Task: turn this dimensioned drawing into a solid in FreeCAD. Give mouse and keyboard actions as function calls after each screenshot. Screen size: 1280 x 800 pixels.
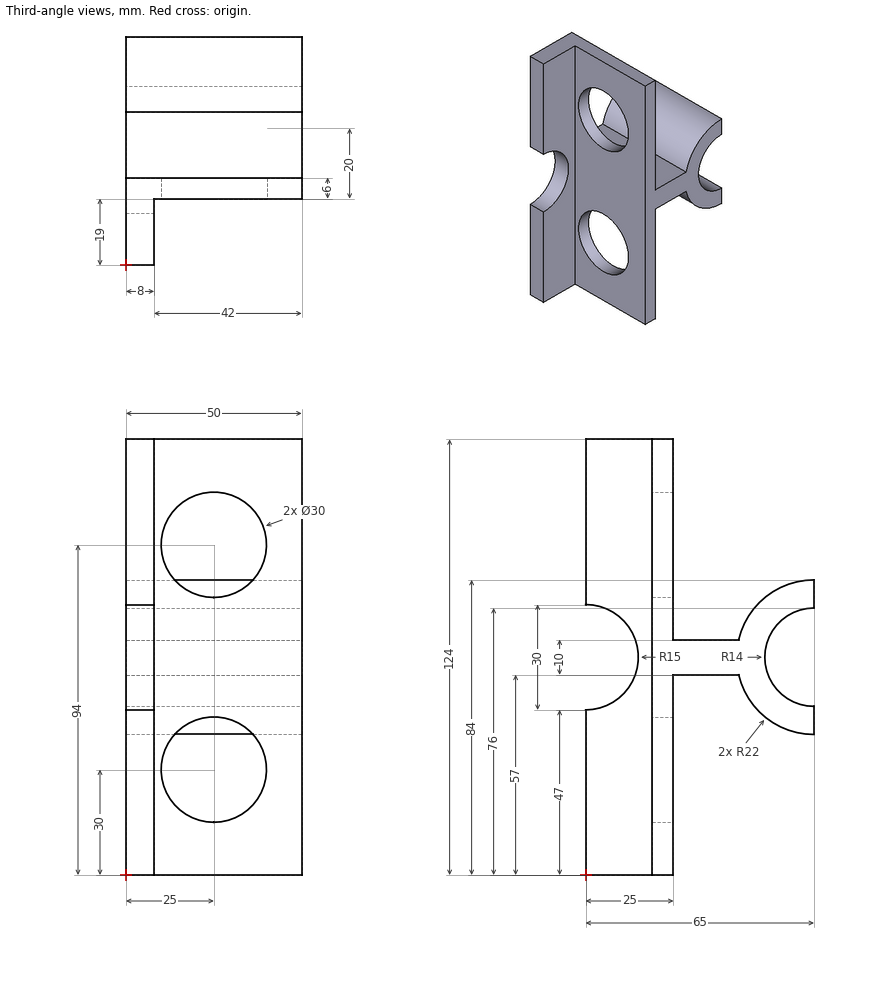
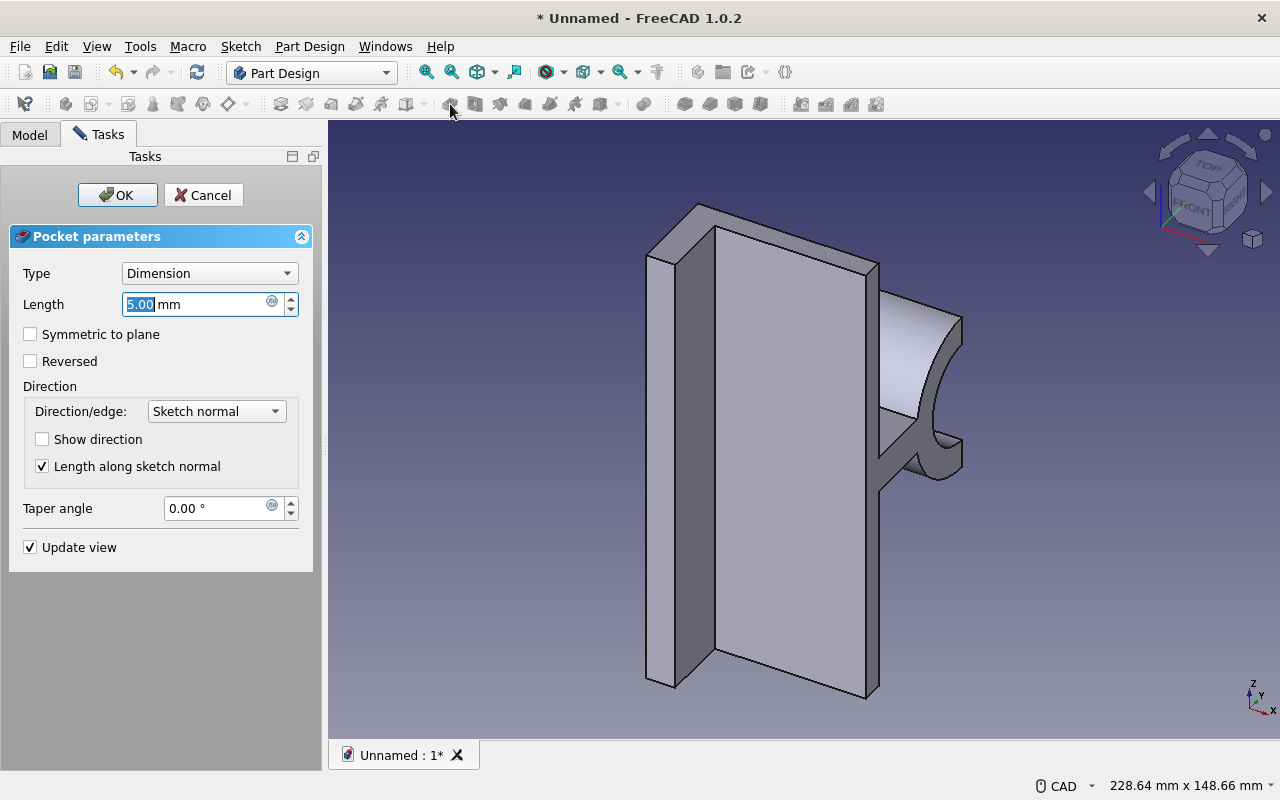
text(50)
key(Tab)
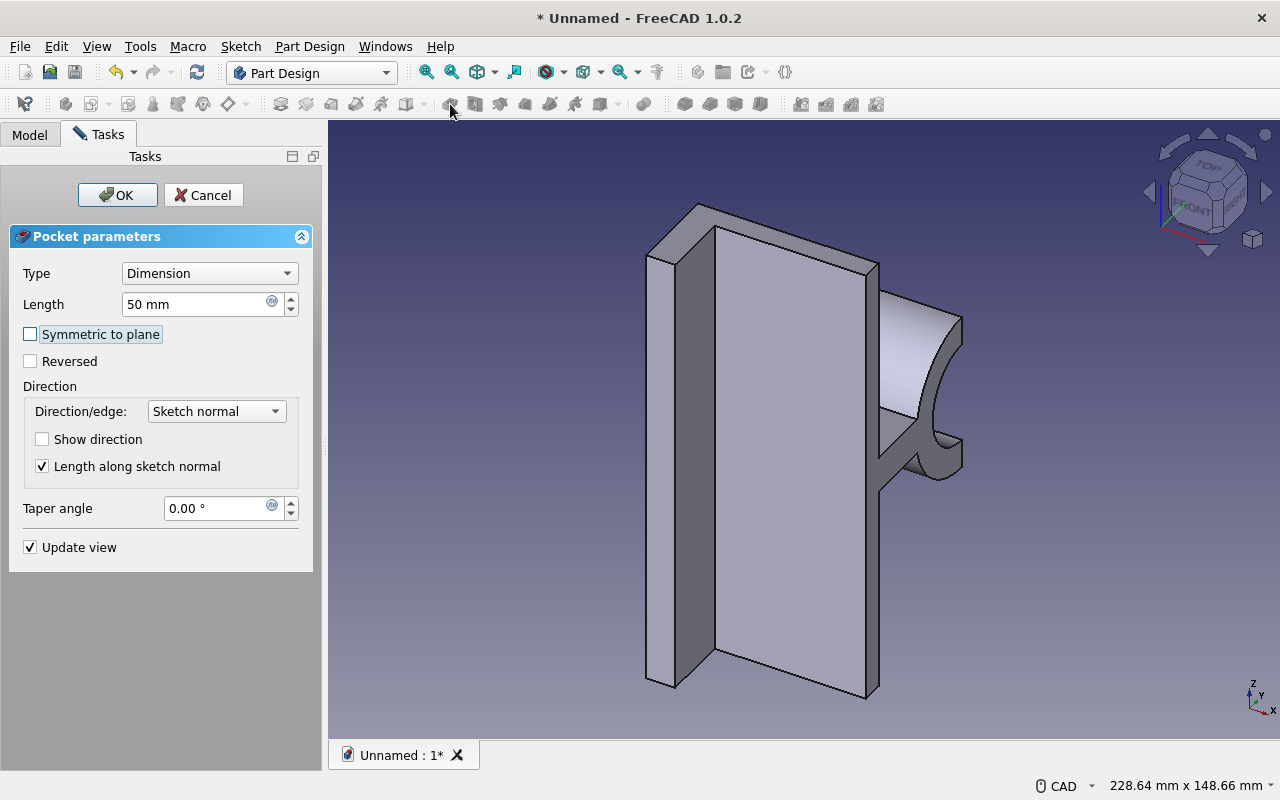
click(31, 361)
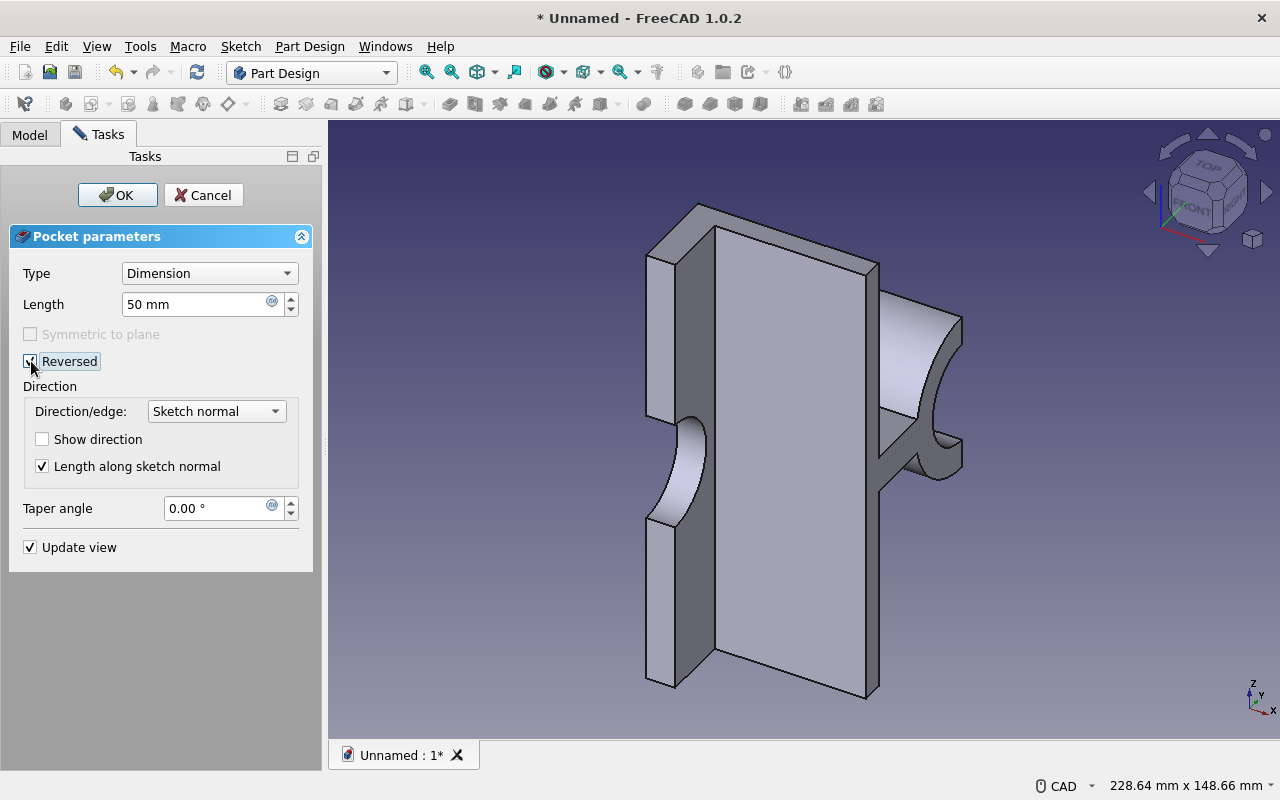
click(118, 195)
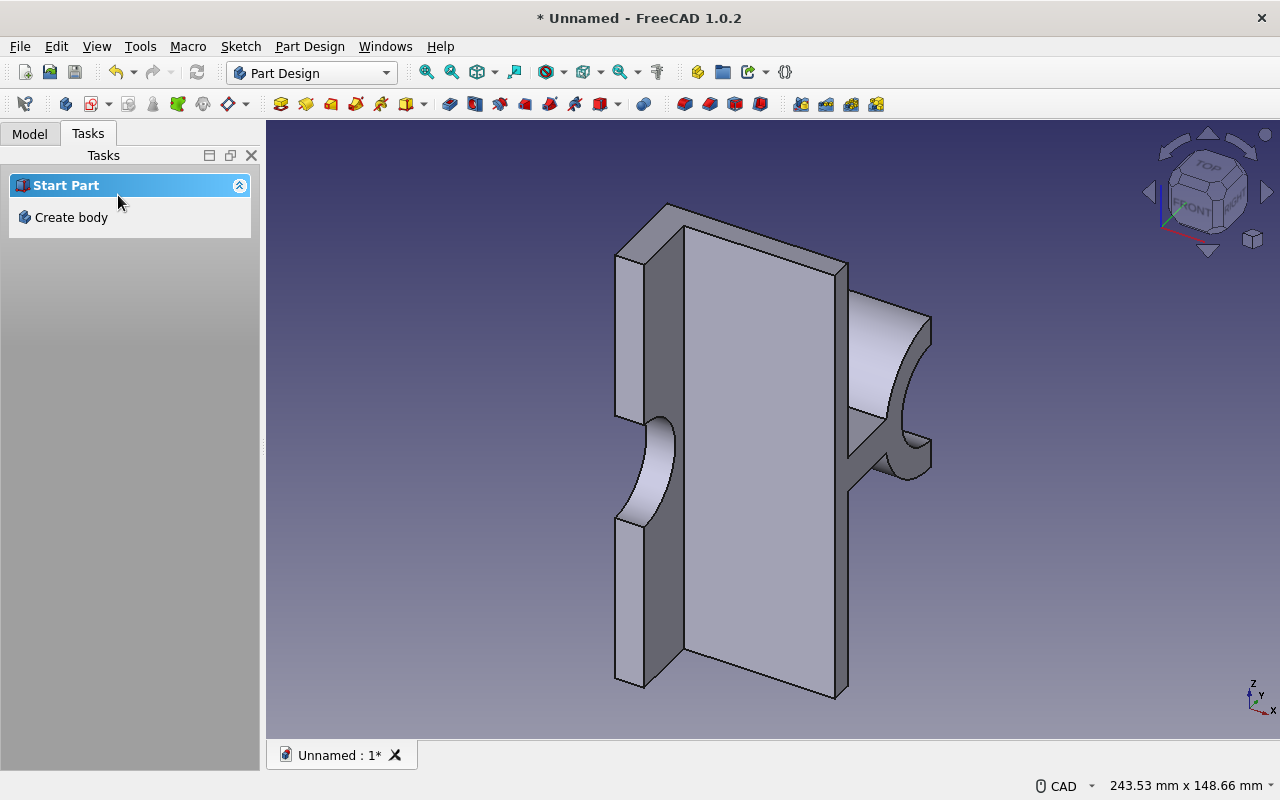
click(759, 340)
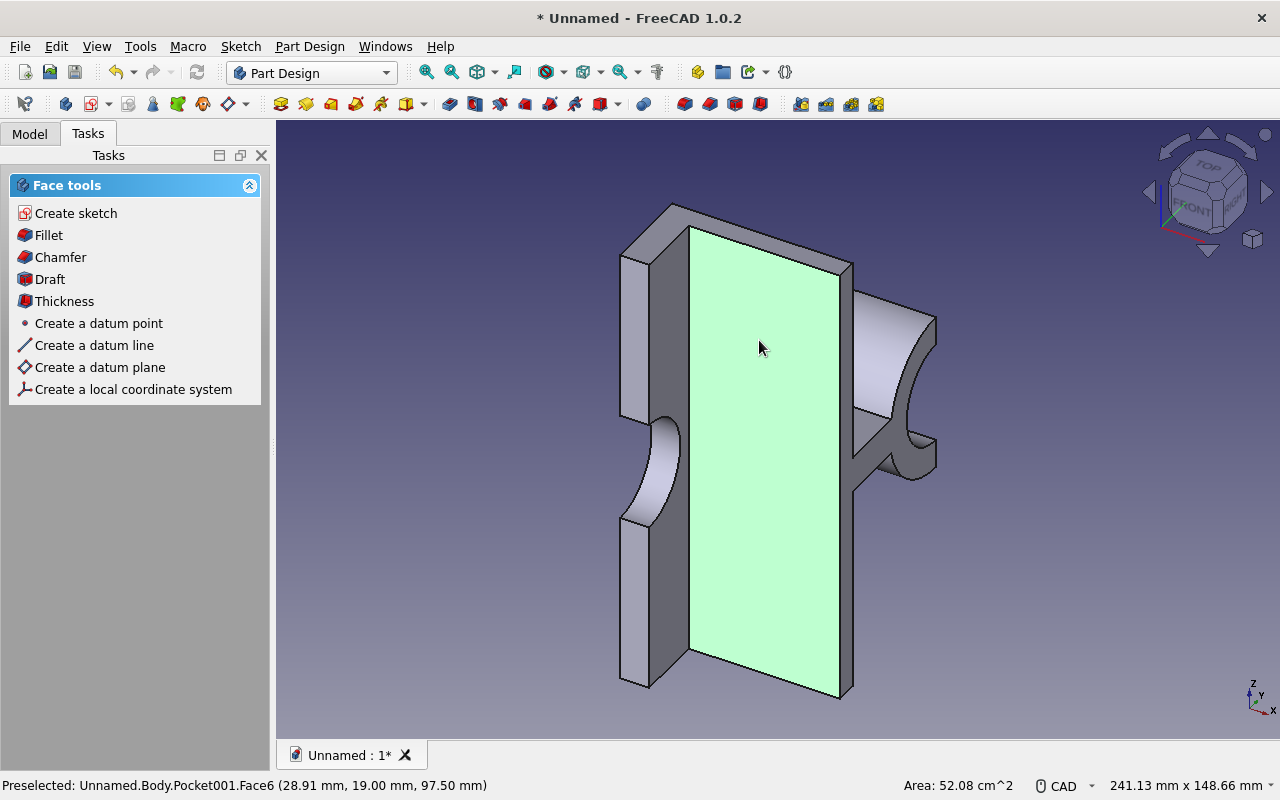
click(90, 104)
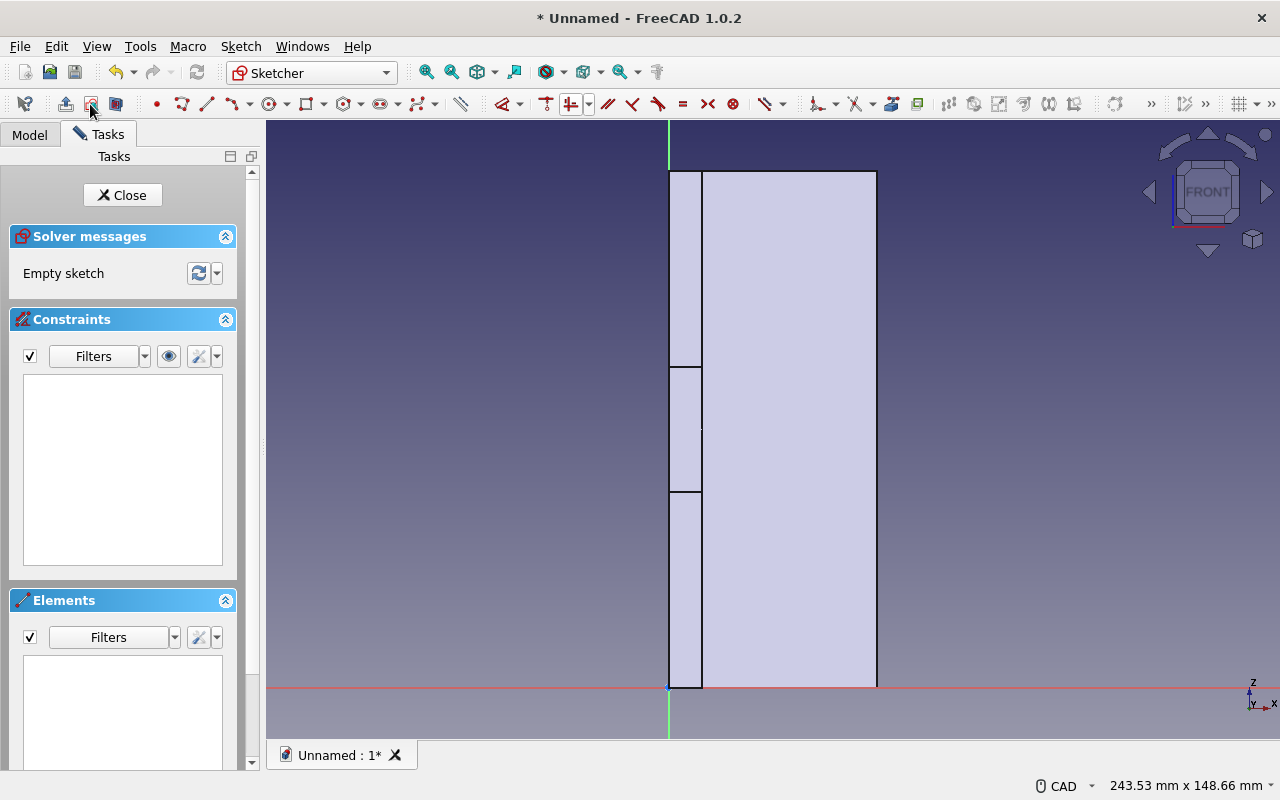
scroll(489, 288, down, 1)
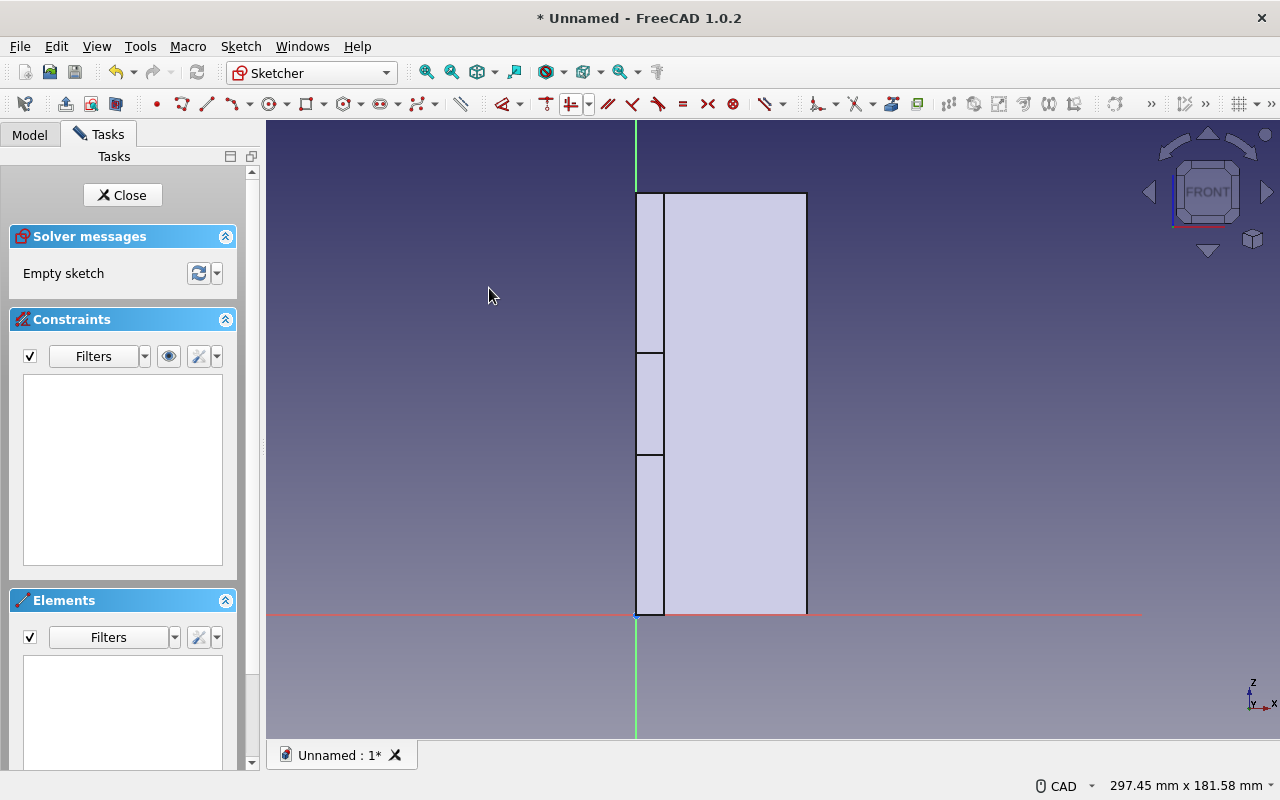
key(g)
key(c)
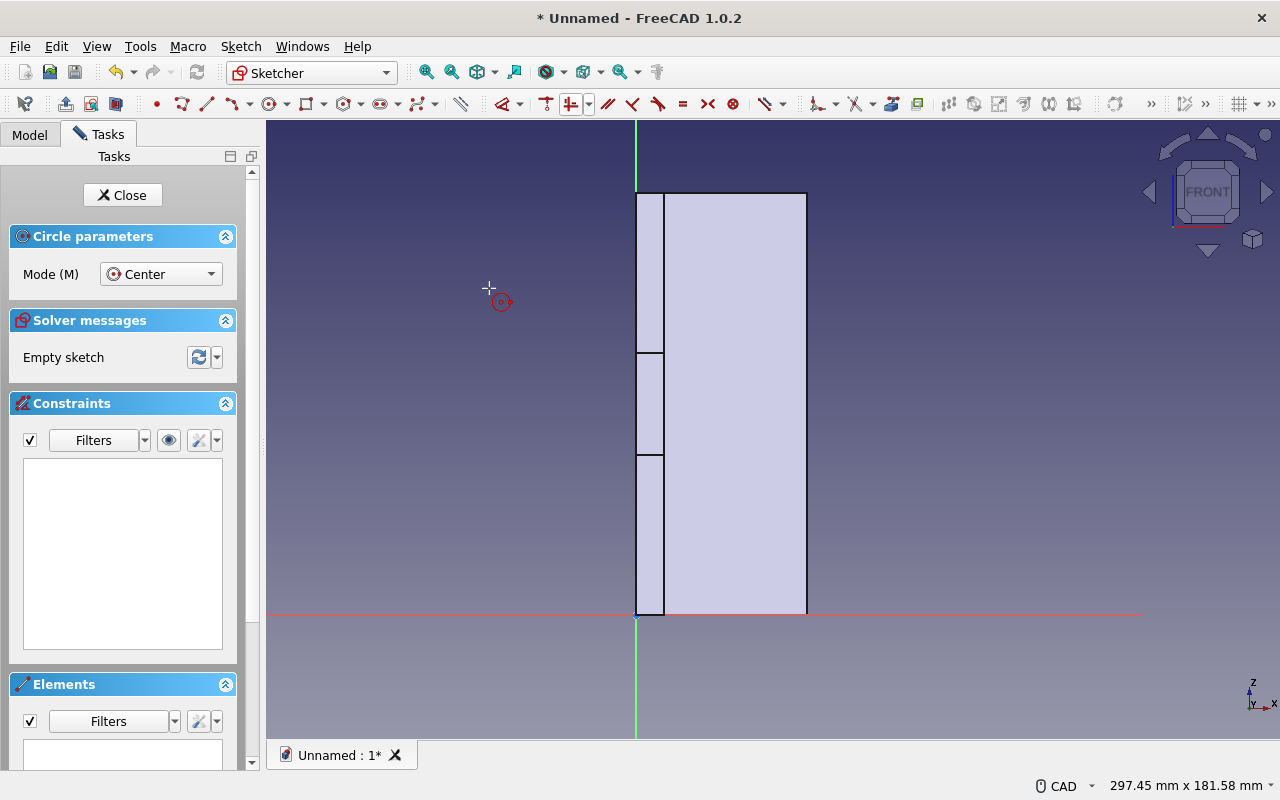
click(722, 295)
click(758, 259)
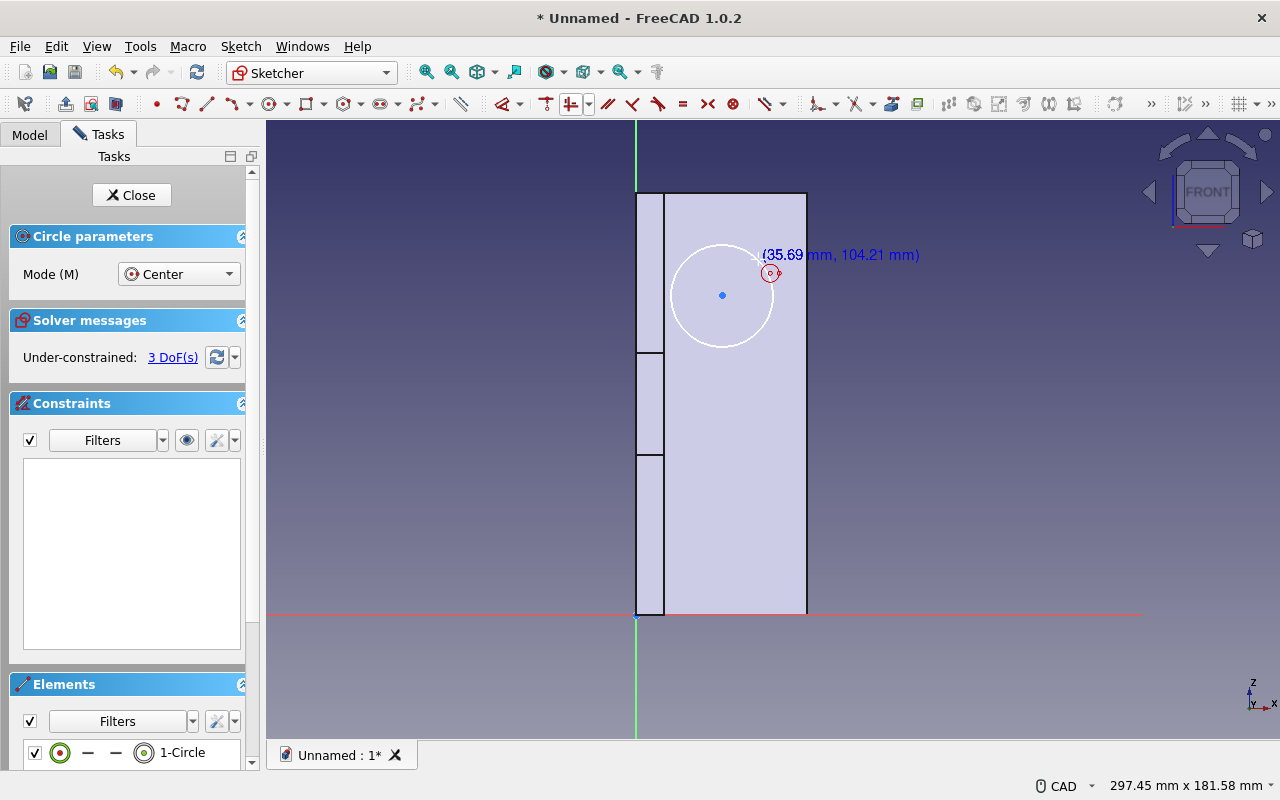
click(722, 513)
click(758, 477)
key(Escape)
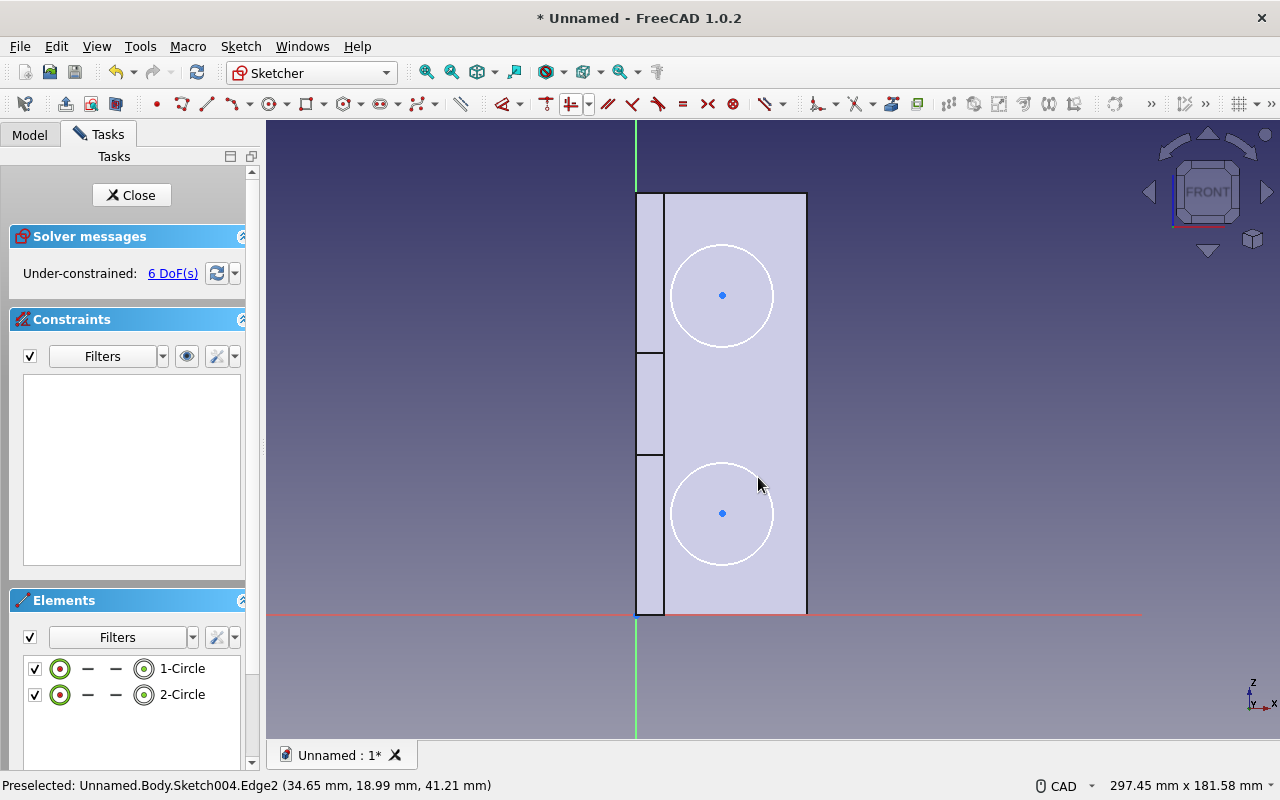
click(758, 260)